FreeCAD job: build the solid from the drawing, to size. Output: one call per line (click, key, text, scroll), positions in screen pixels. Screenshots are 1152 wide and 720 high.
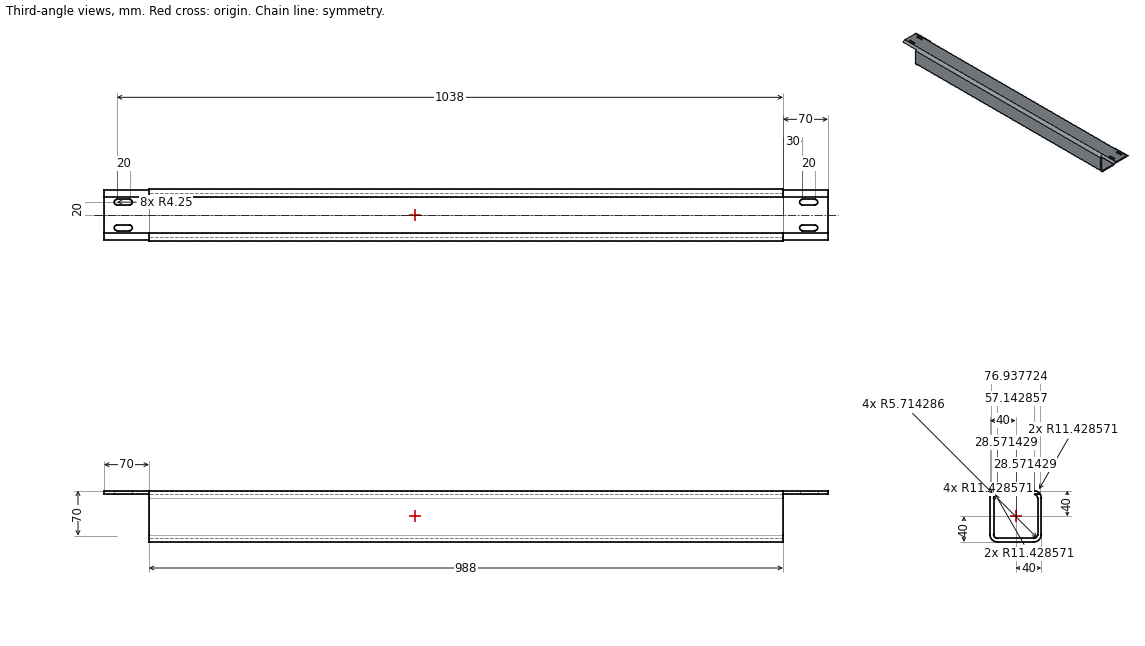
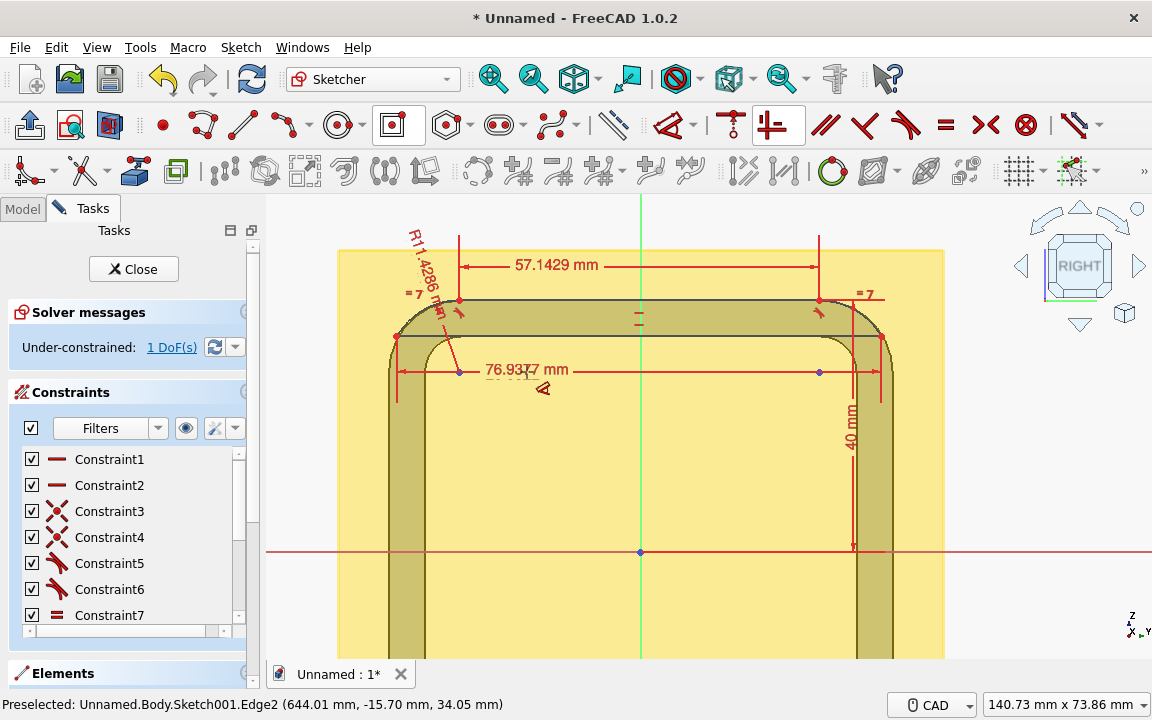
click(819, 300)
click(730, 586)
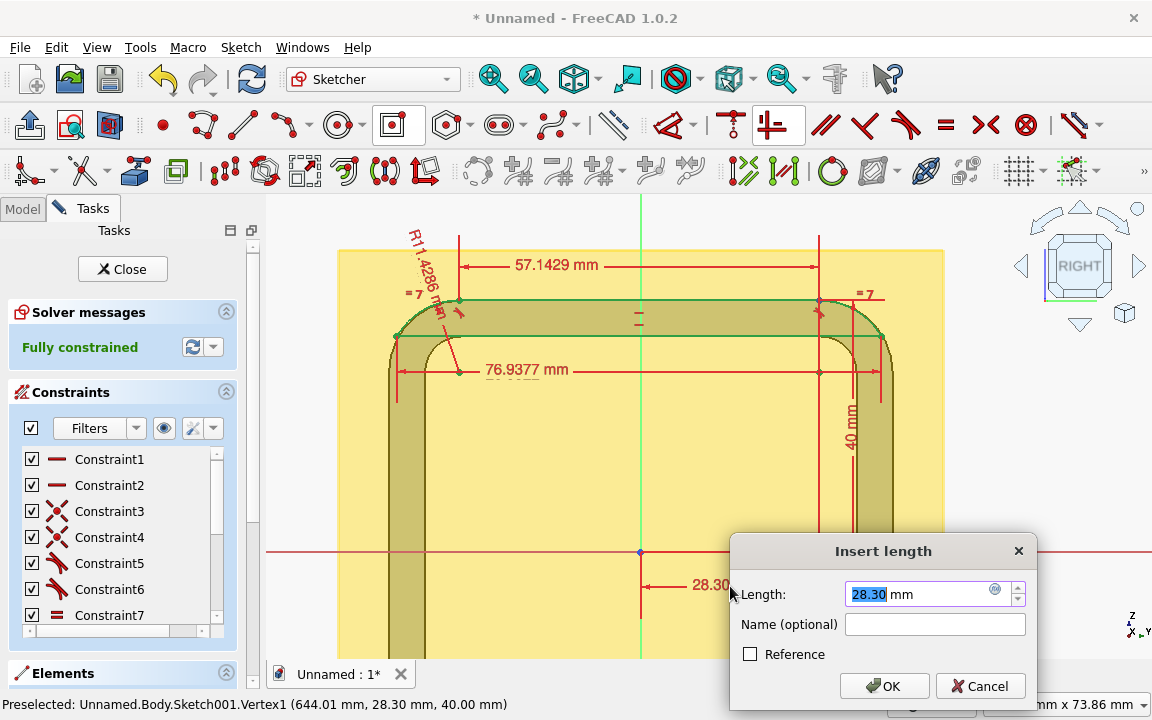
text(28.571429)
key(Return)
key(Escape)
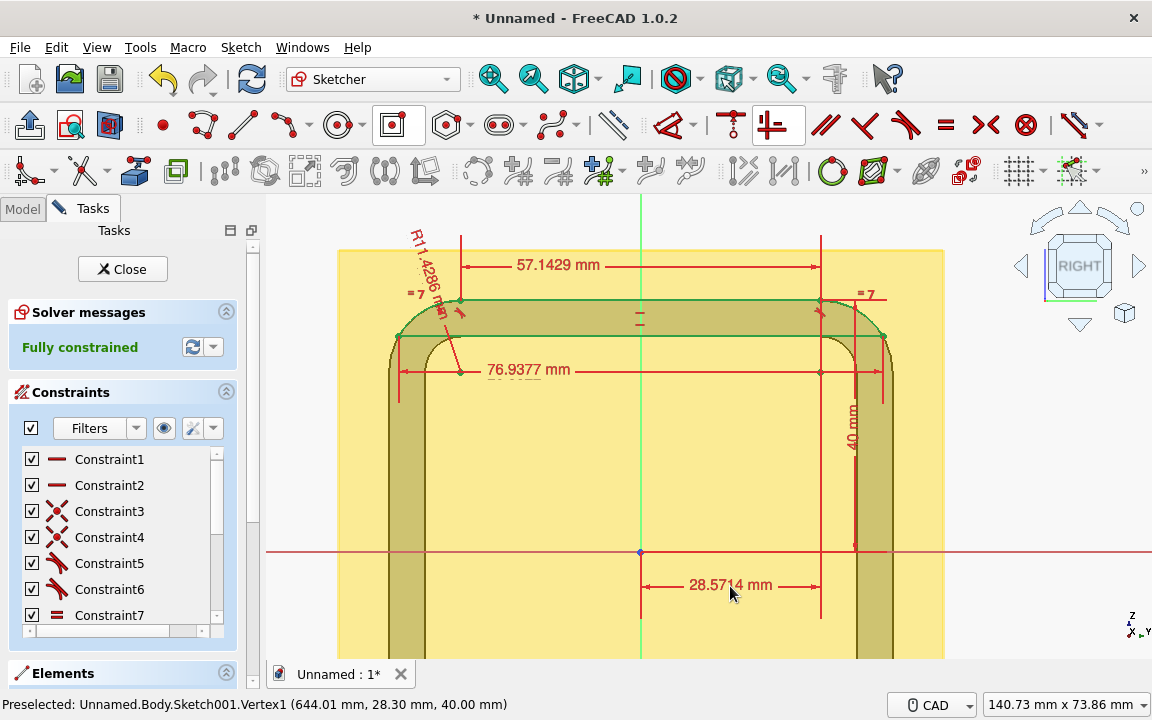
click(123, 269)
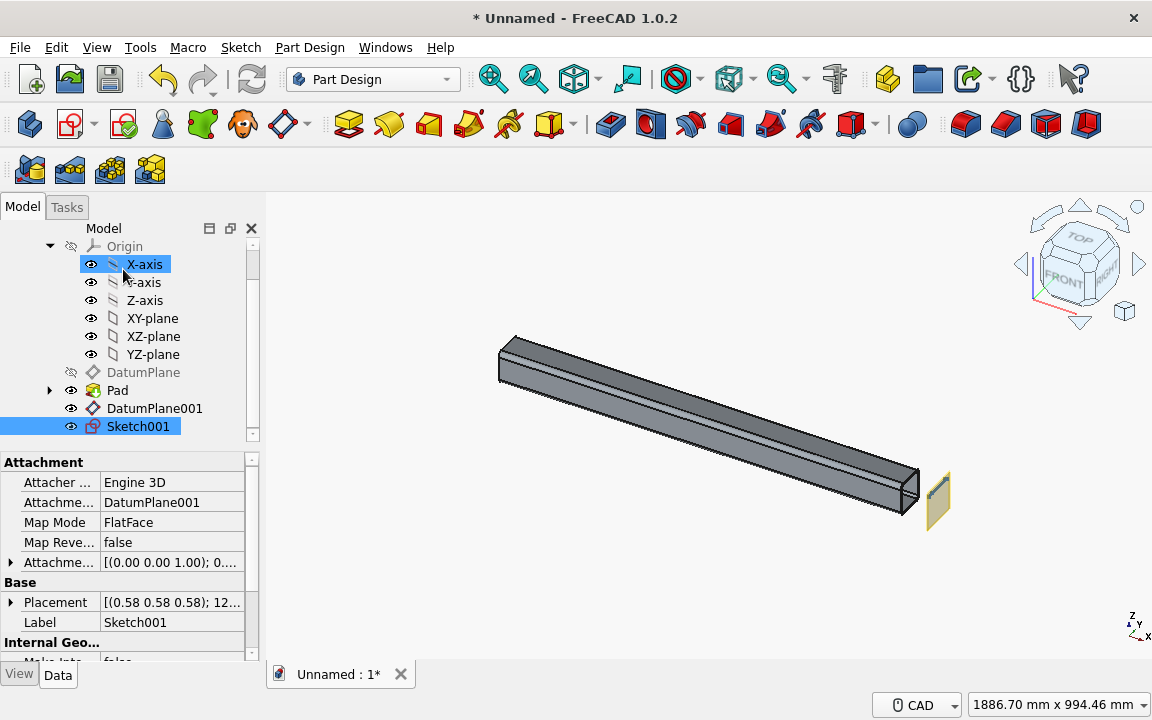
click(350, 124)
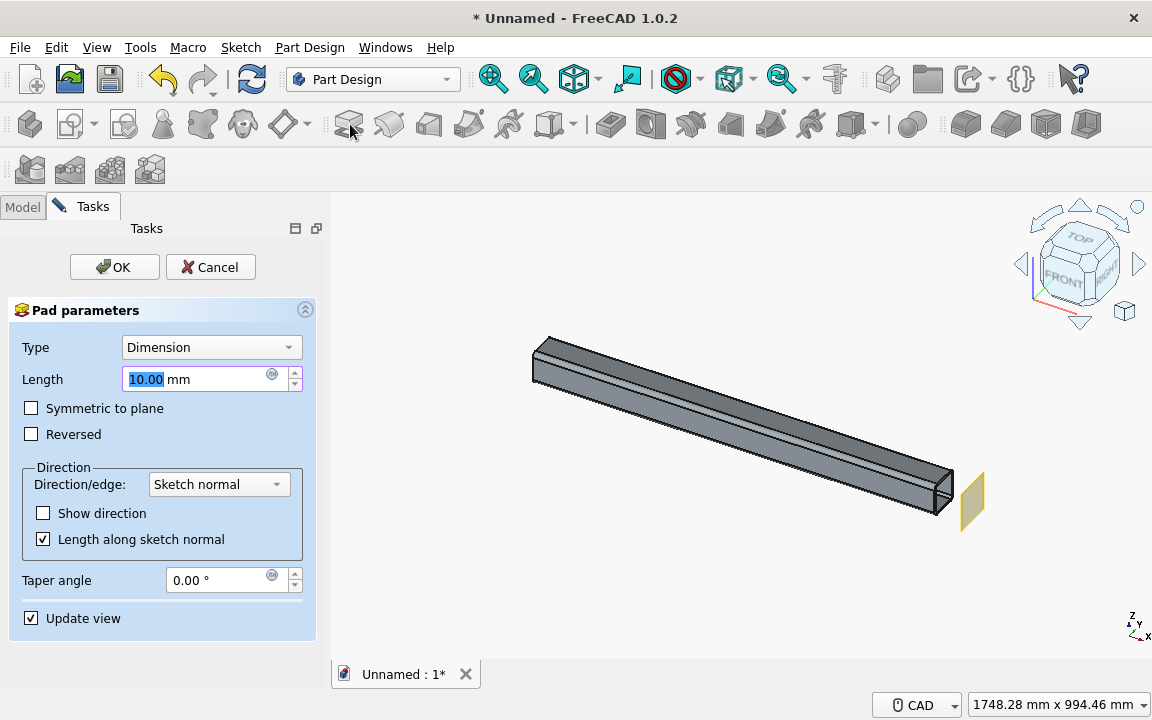
text(70)
key(Tab)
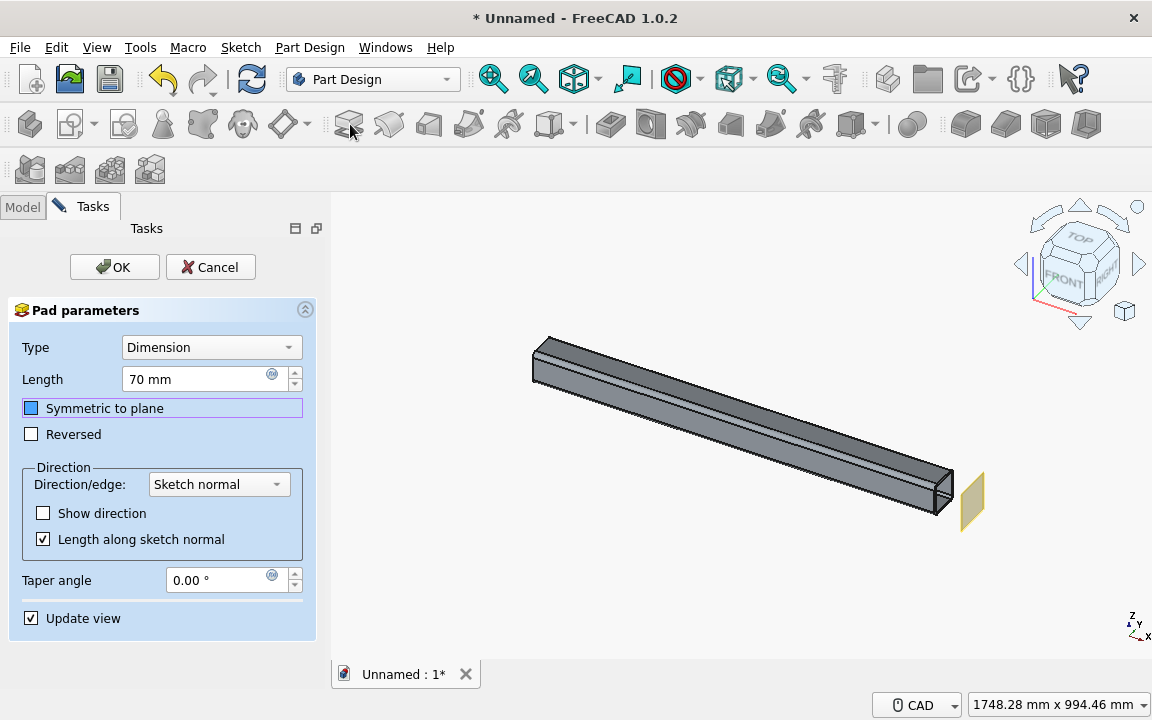
click(30, 434)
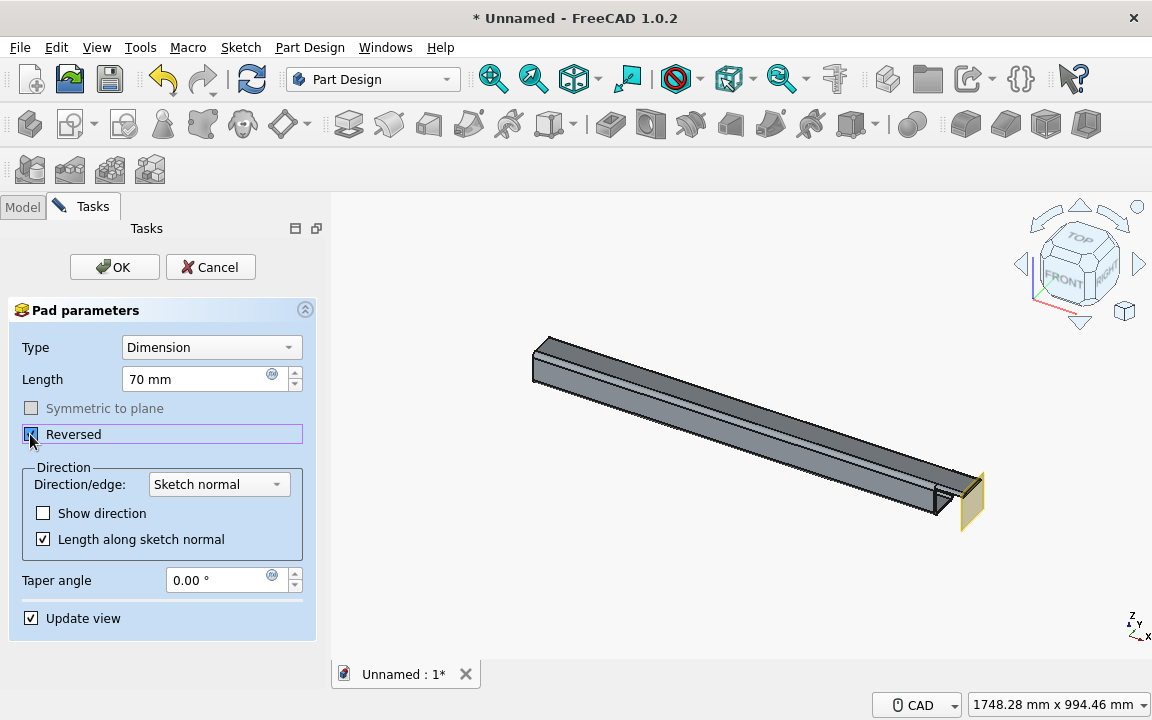
click(115, 267)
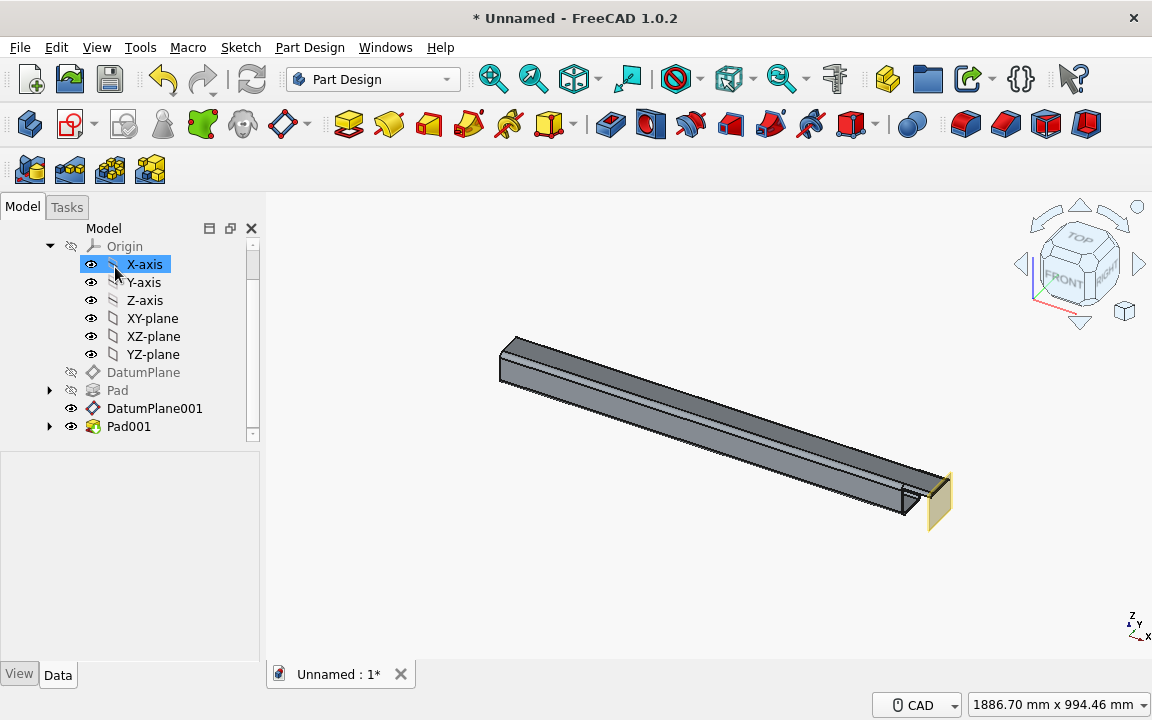
click(116, 408)
key(space)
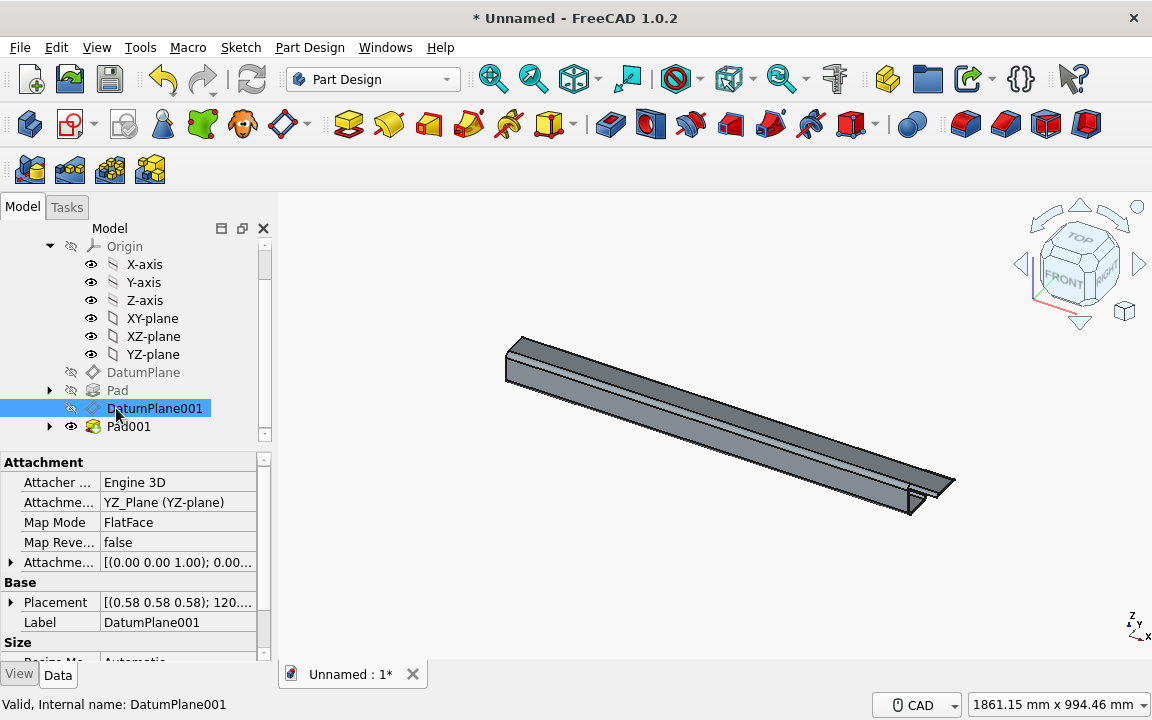
key(6)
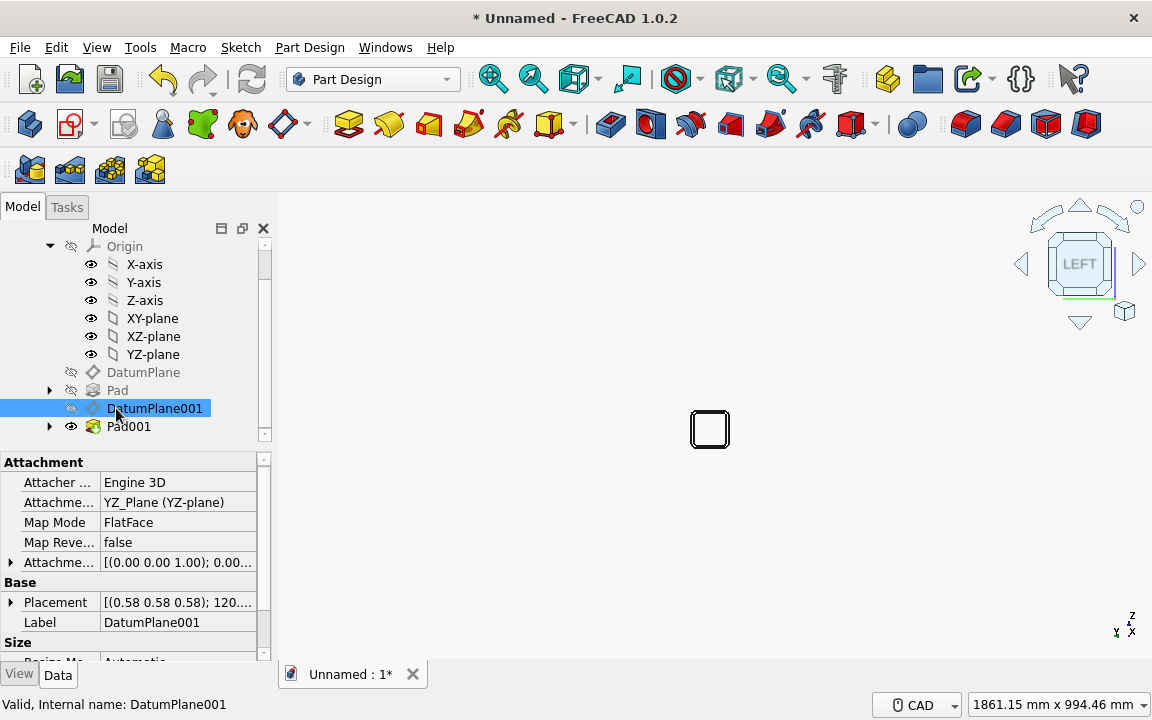
key(v)
key(f)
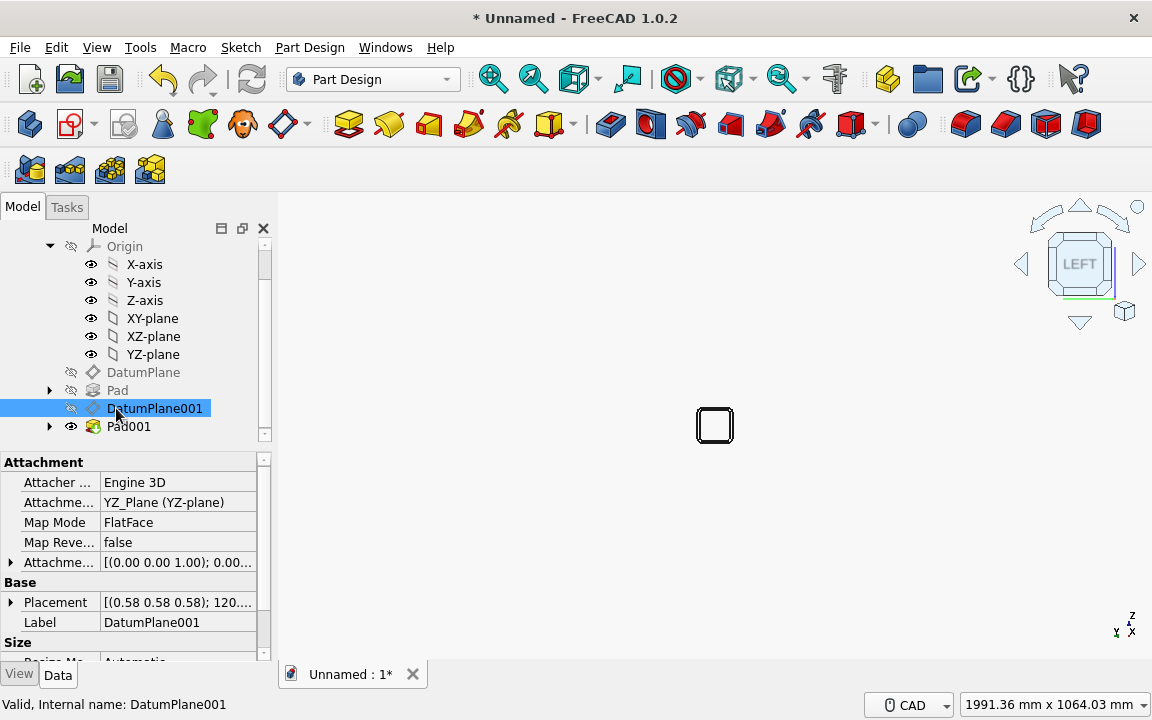
scroll(730, 409, up, 13)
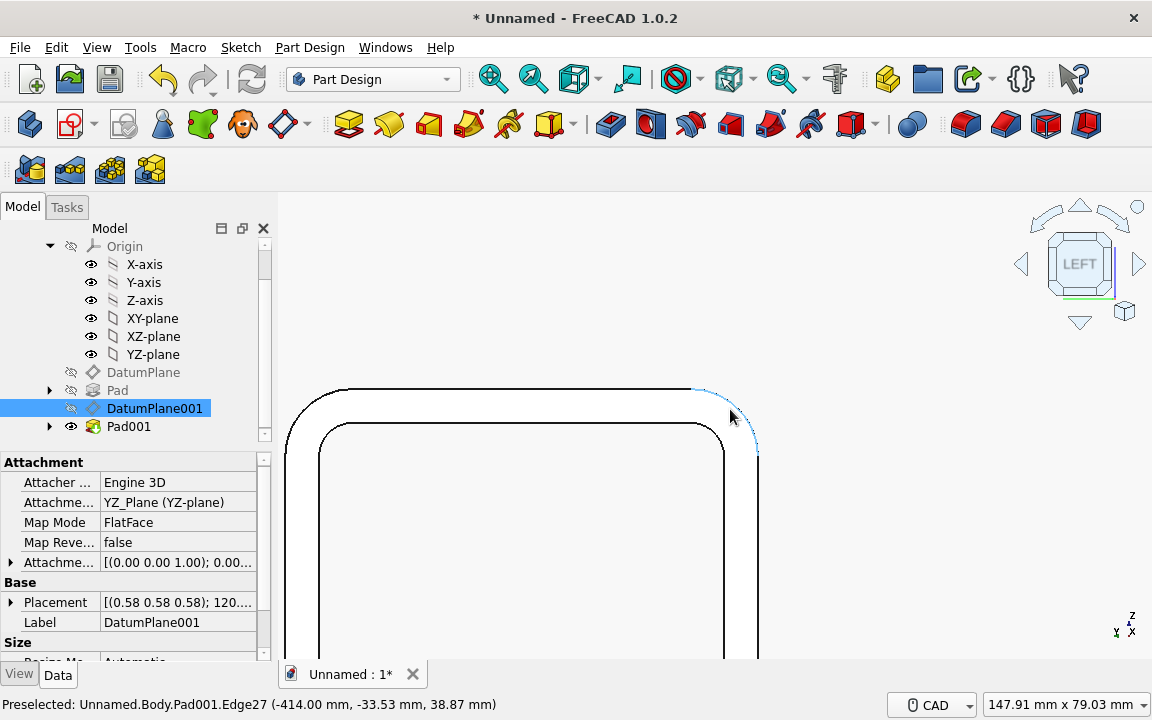
click(724, 422)